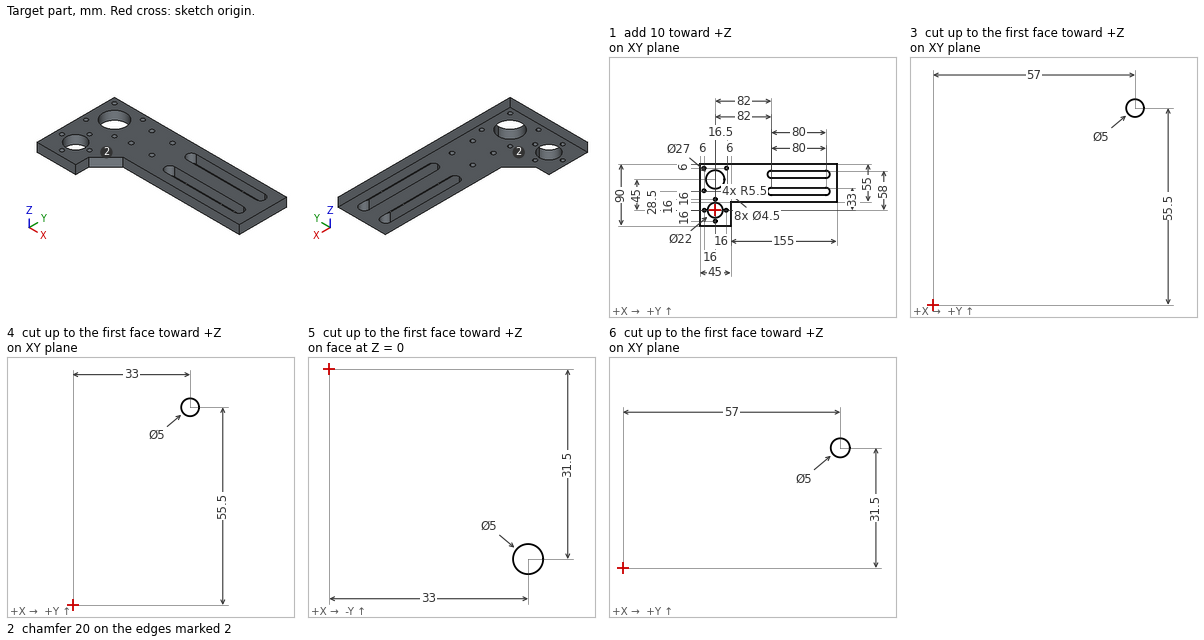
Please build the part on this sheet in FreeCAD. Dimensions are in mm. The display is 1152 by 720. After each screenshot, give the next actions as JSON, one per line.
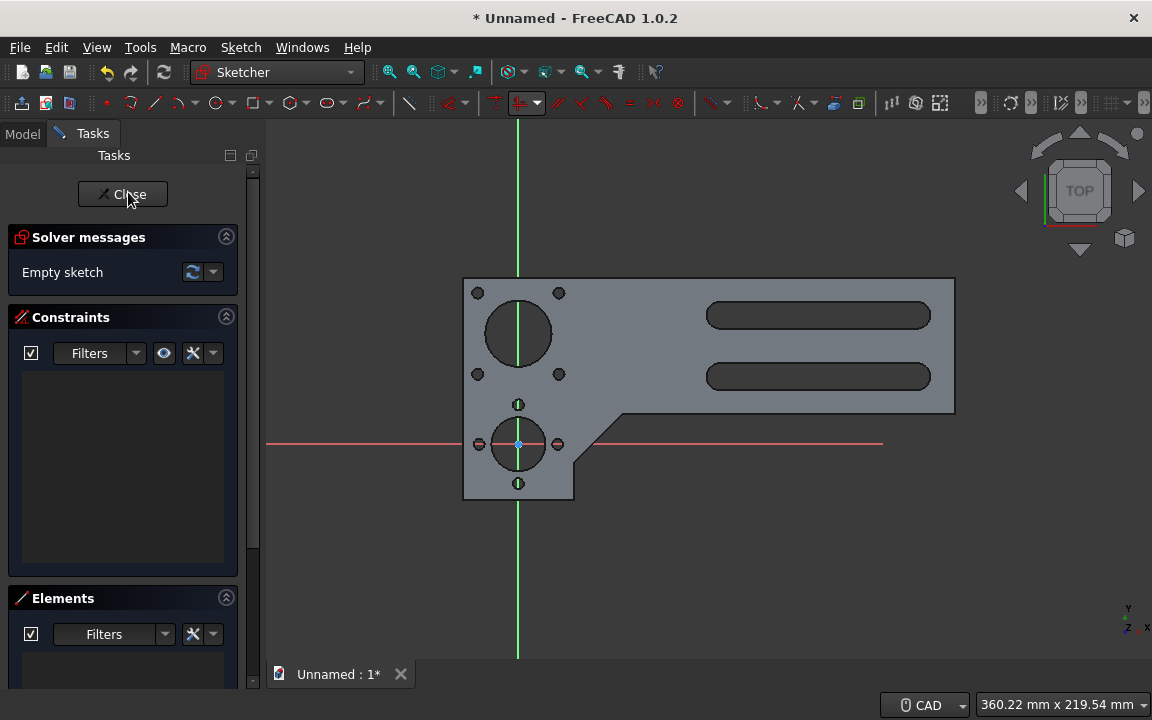
{"action": "key", "text": "q s"}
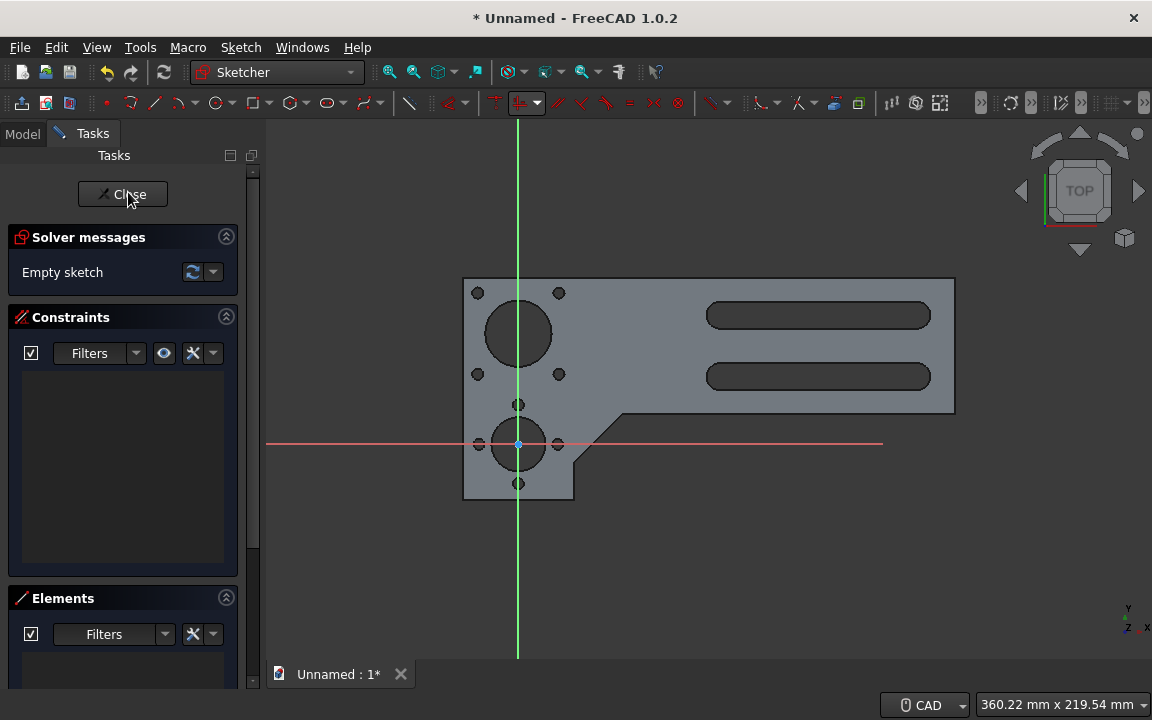
{"action": "scroll", "coordinate": [660, 304], "scroll_direction": "up", "scroll_amount": 15}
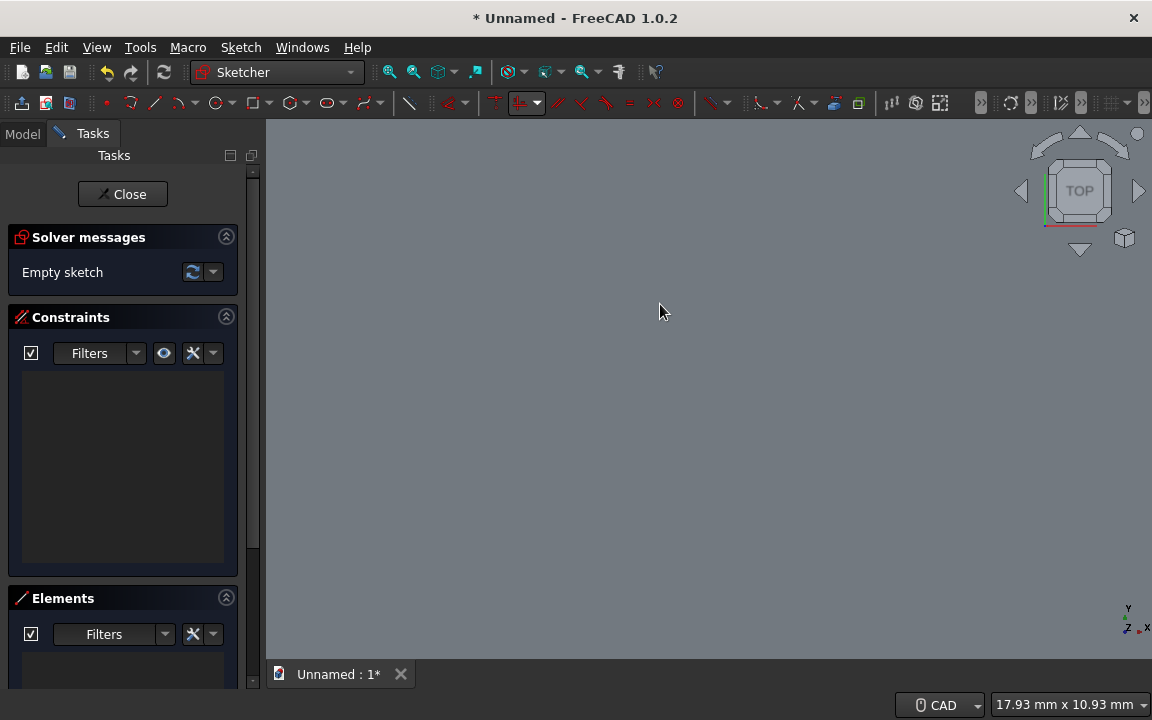
{"action": "scroll", "coordinate": [587, 345], "scroll_direction": "up", "scroll_amount": 2}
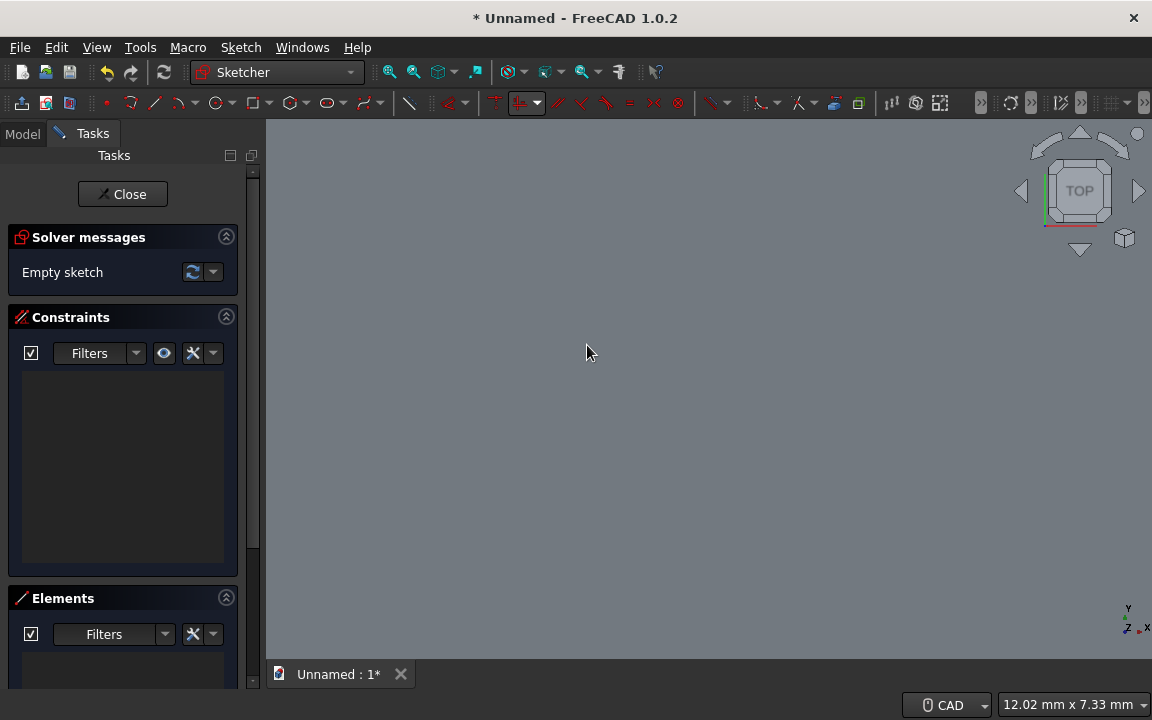
{"action": "key", "text": "g c"}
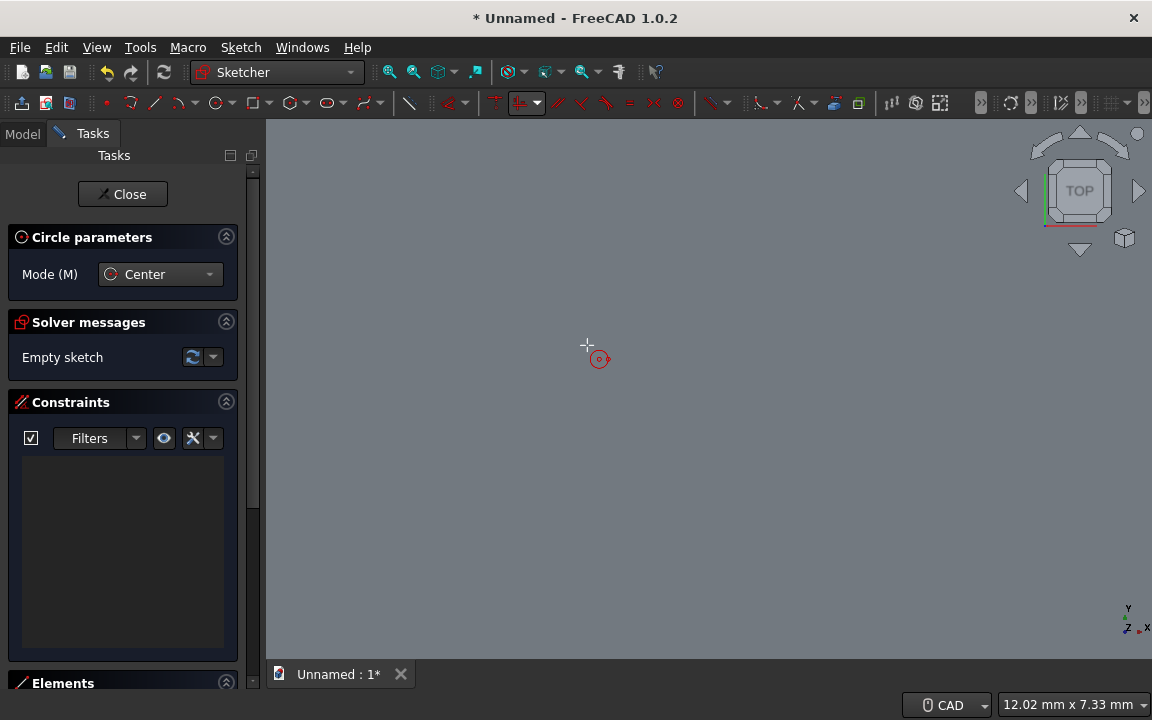
{"action": "left_click", "coordinate": [640, 389]}
{"action": "mouse_move", "coordinate": [771, 258]}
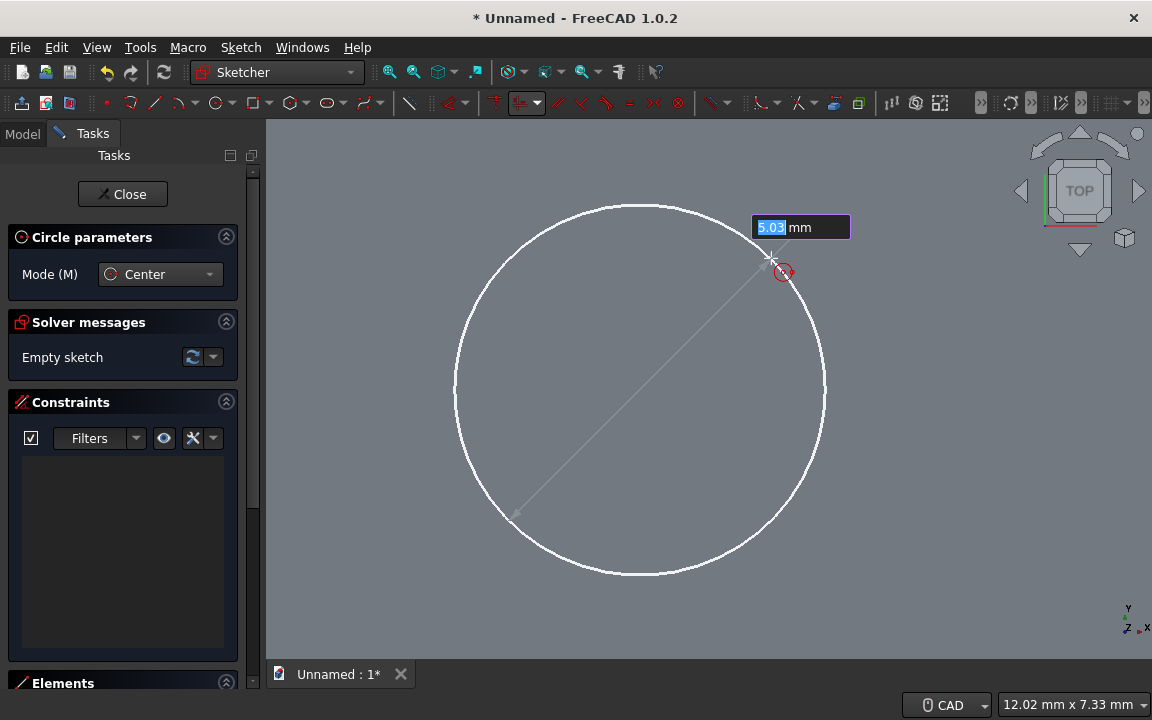
{"action": "type", "text": "5"}
{"action": "key", "text": "Return"}
{"action": "key", "text": "Escape"}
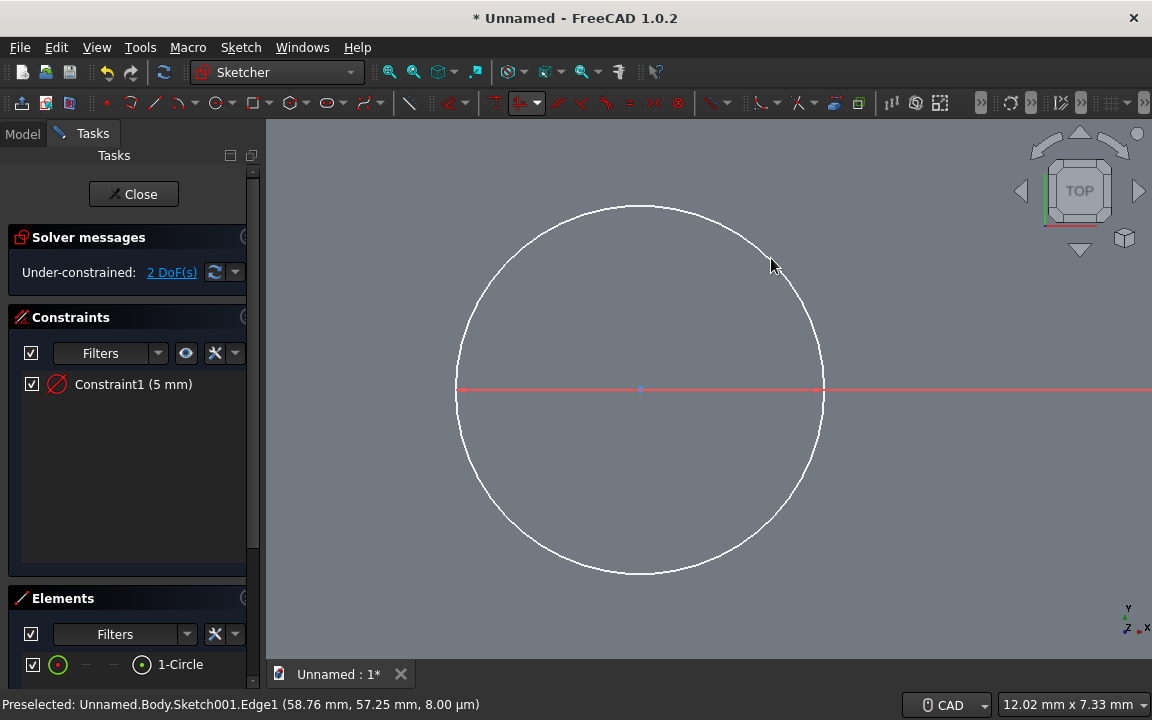
{"action": "left_click", "coordinate": [448, 104]}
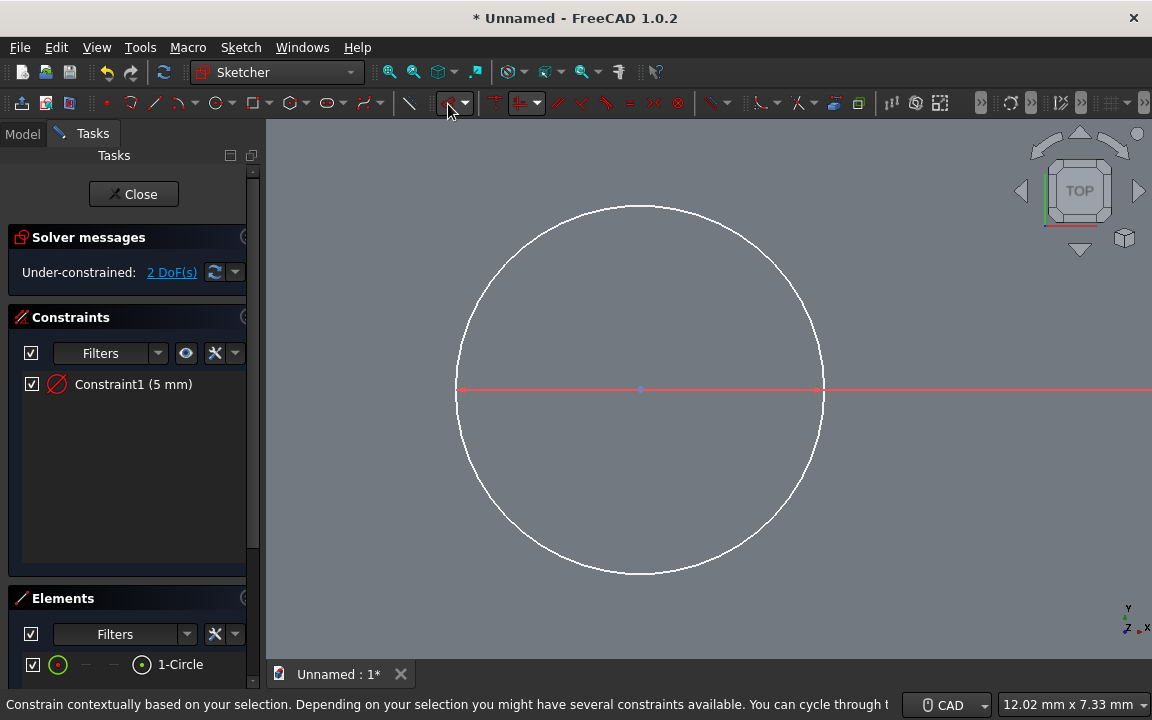
{"action": "left_click", "coordinate": [640, 390]}
{"action": "left_click", "coordinate": [387, 356]}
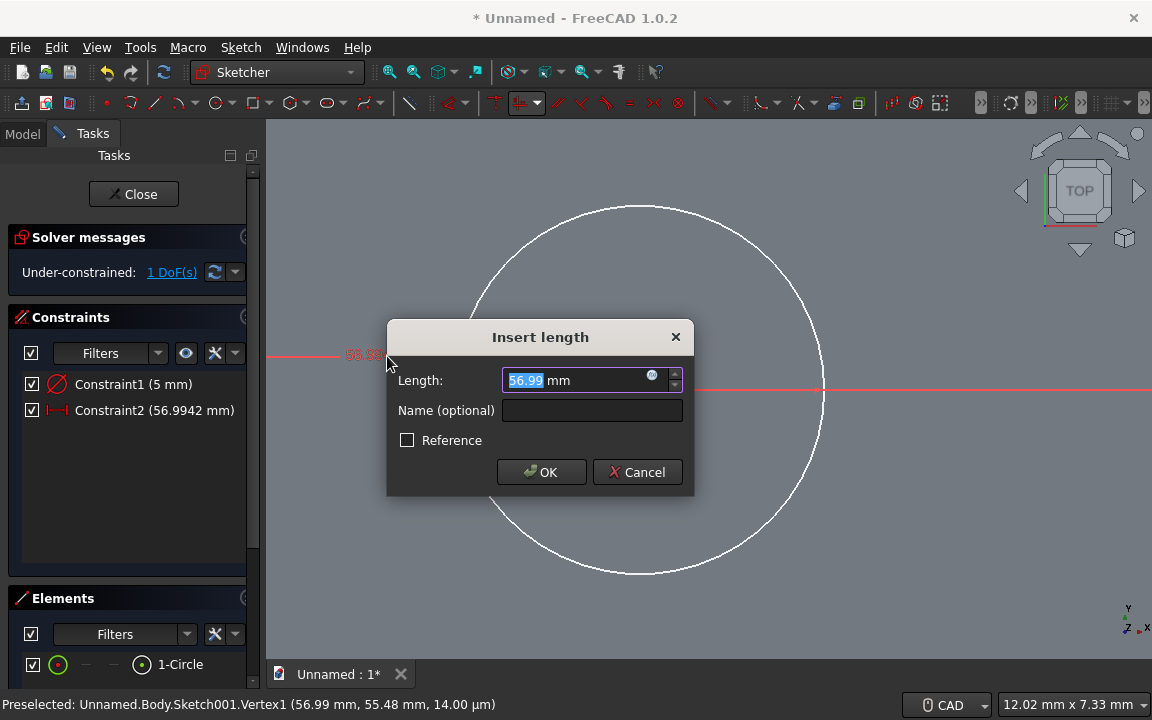
{"action": "type", "text": "57"}
{"action": "key", "text": "Return"}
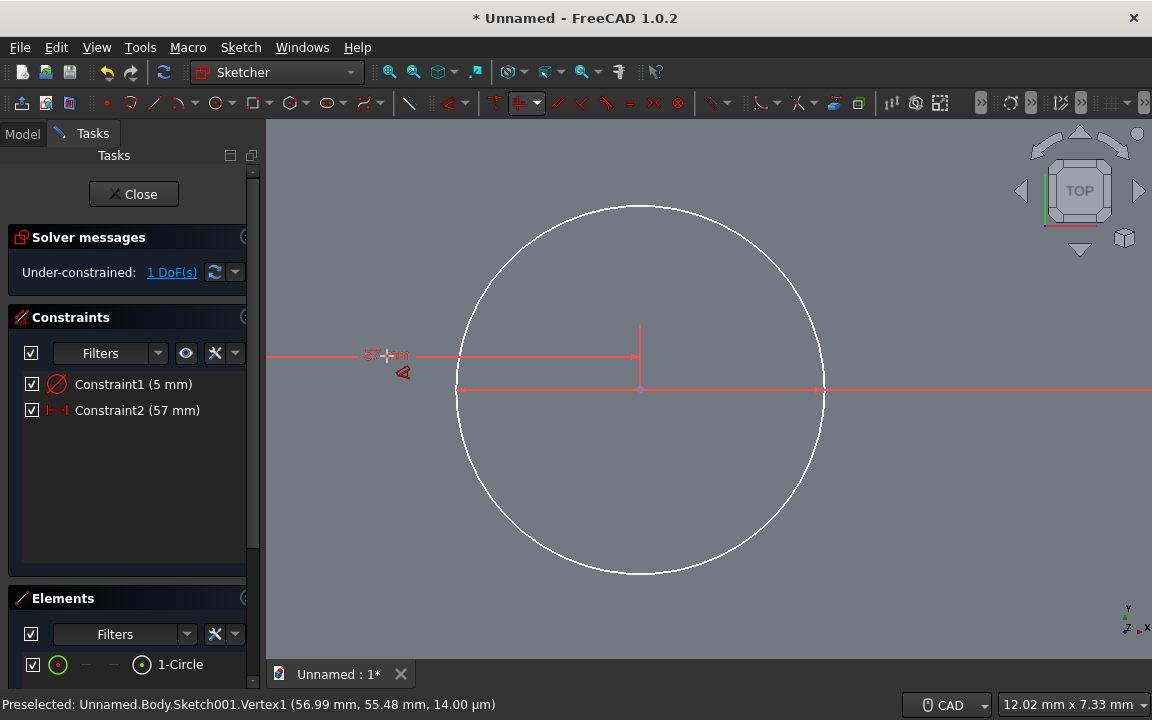
{"action": "left_click", "coordinate": [640, 390]}
{"action": "left_click", "coordinate": [674, 511]}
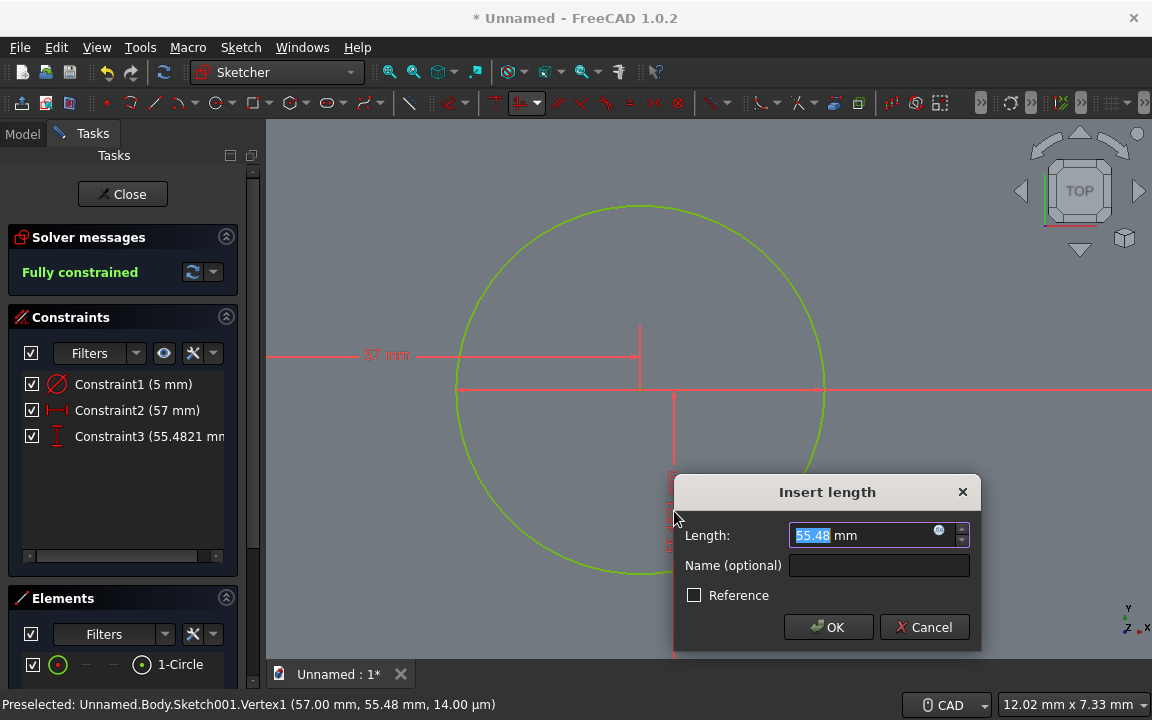
{"action": "type", "text": "55.5"}
{"action": "key", "text": "Return"}
{"action": "key", "text": "Escape"}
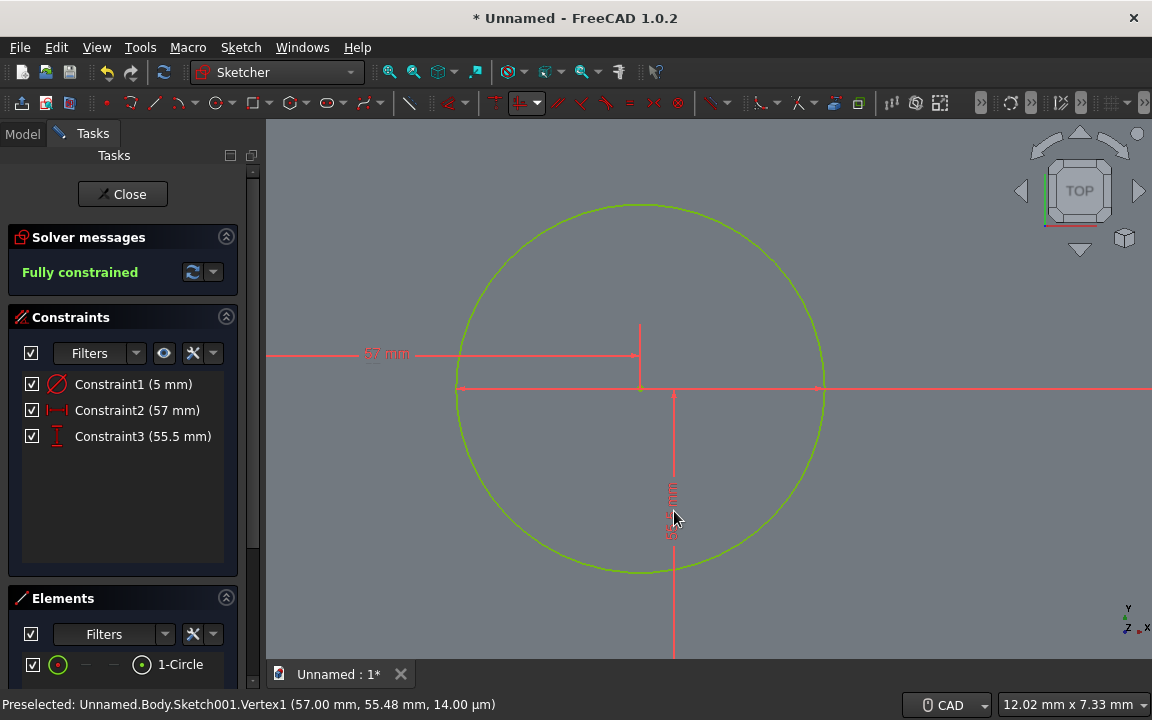
{"action": "left_click", "coordinate": [123, 194]}